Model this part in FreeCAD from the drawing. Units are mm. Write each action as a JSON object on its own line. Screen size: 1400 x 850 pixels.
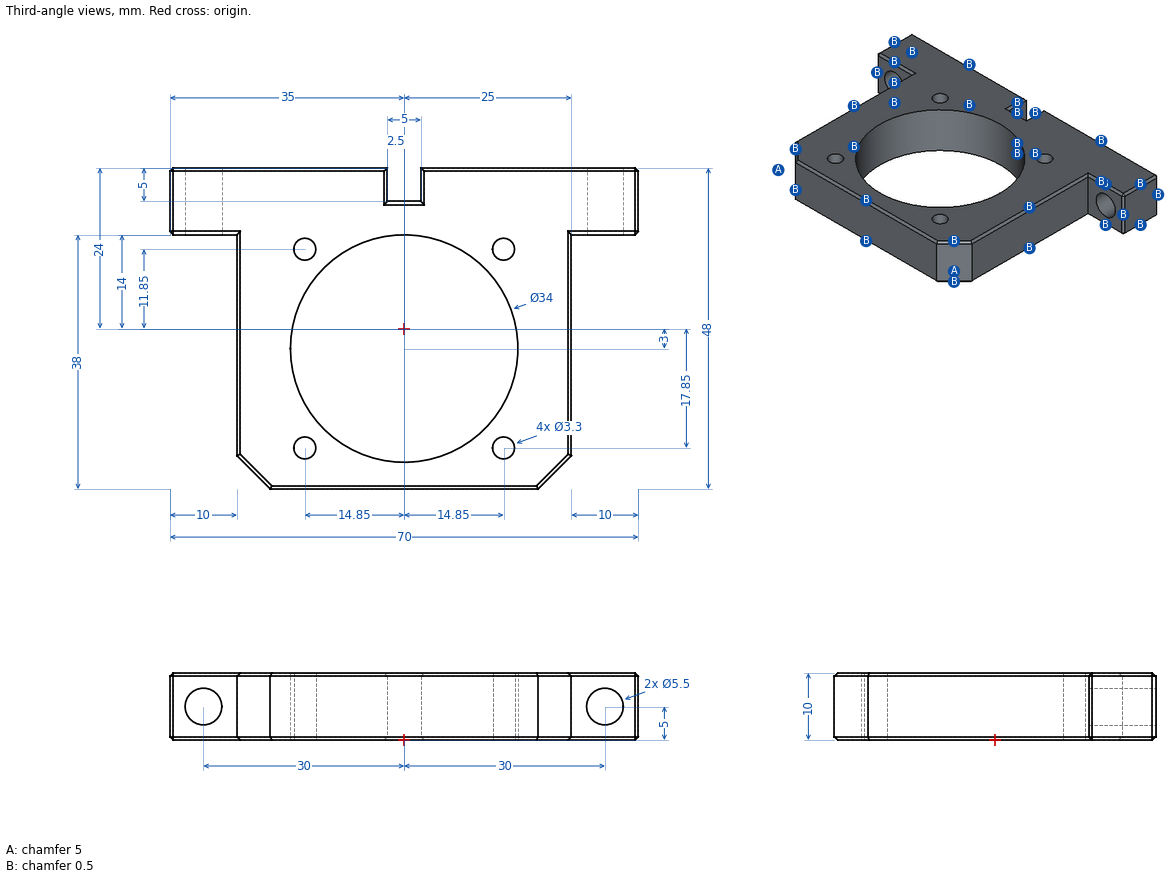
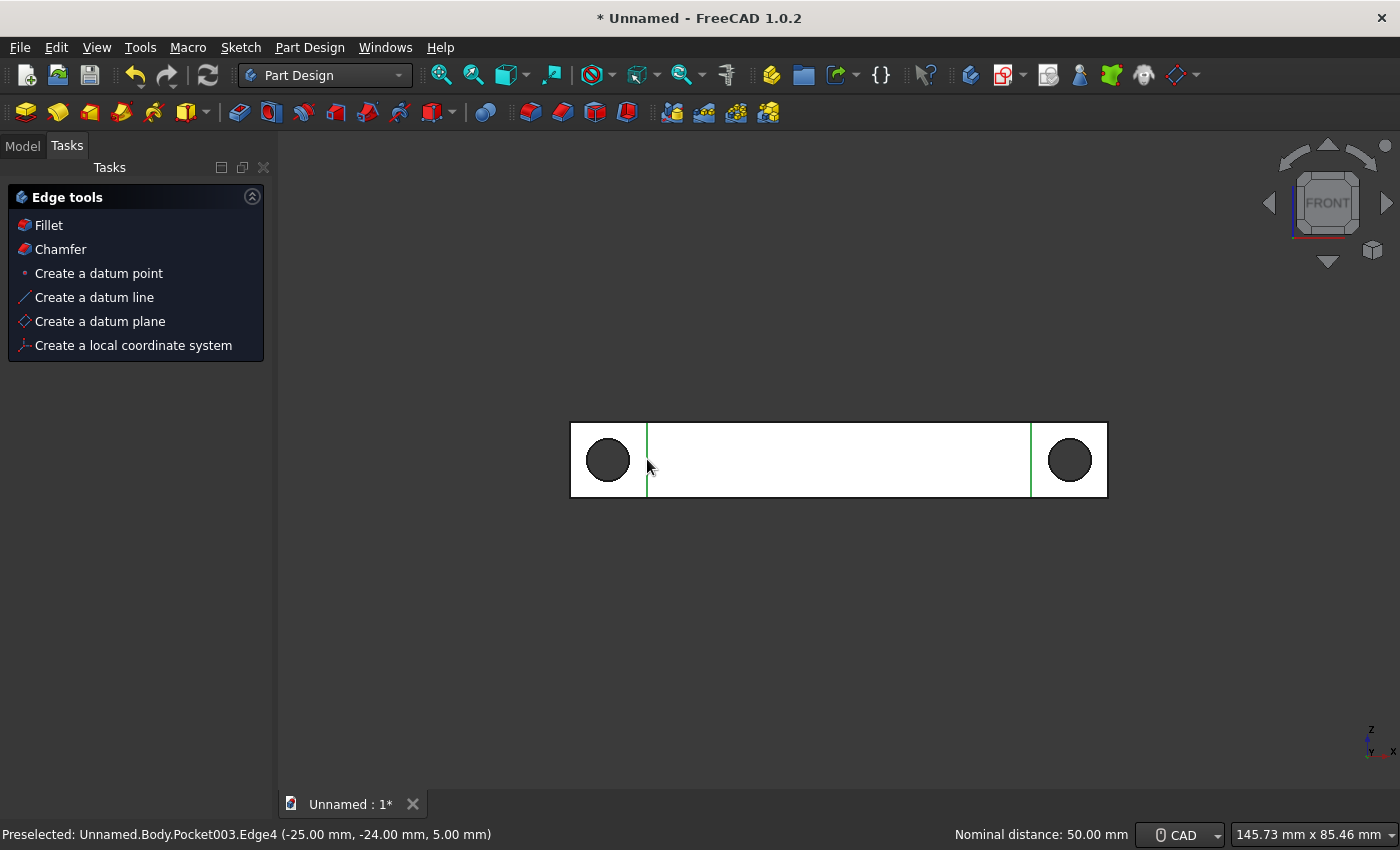
{"action": "left_click", "coordinate": [564, 112]}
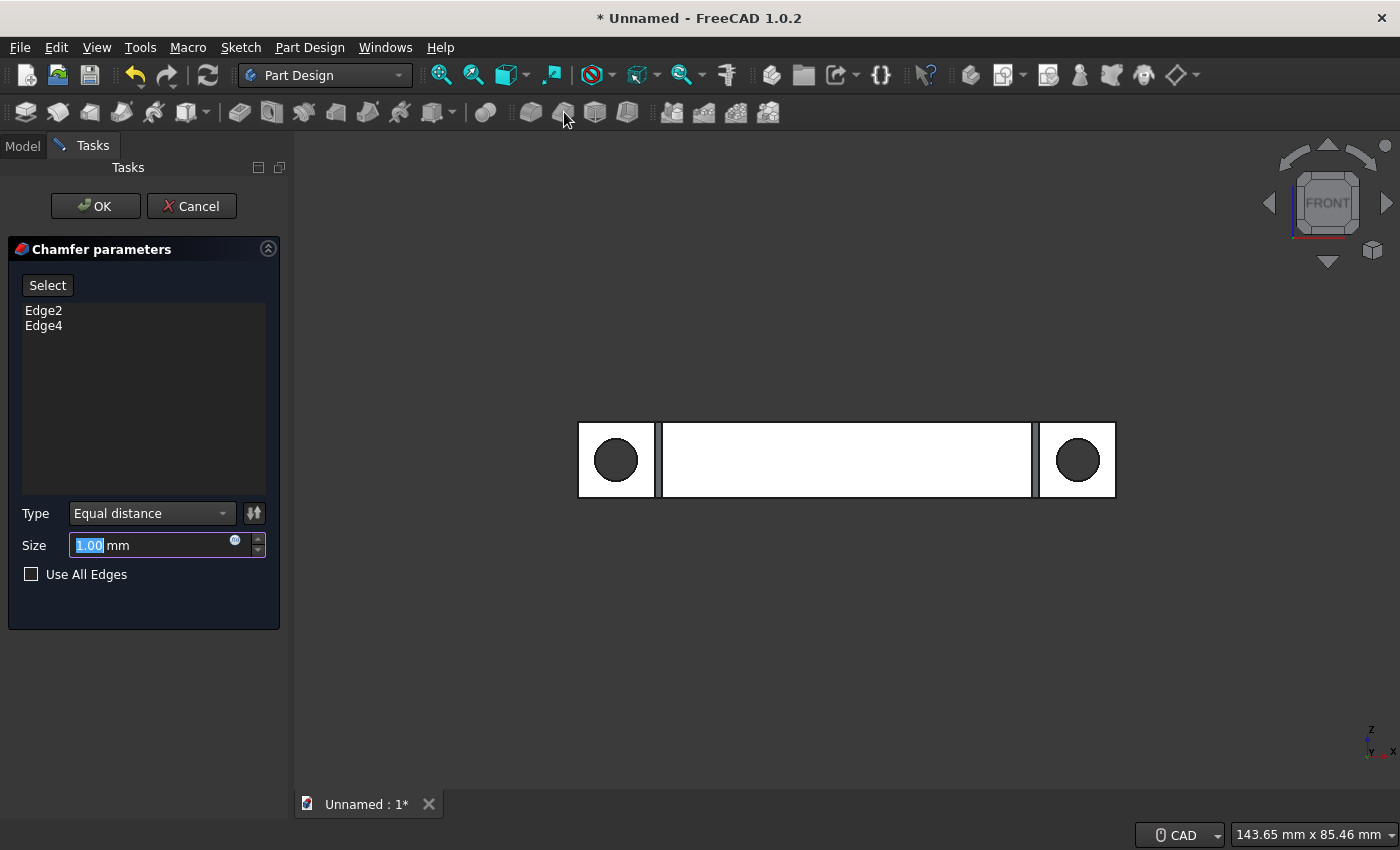
{"action": "type", "text": "5"}
{"action": "key", "text": "Tab"}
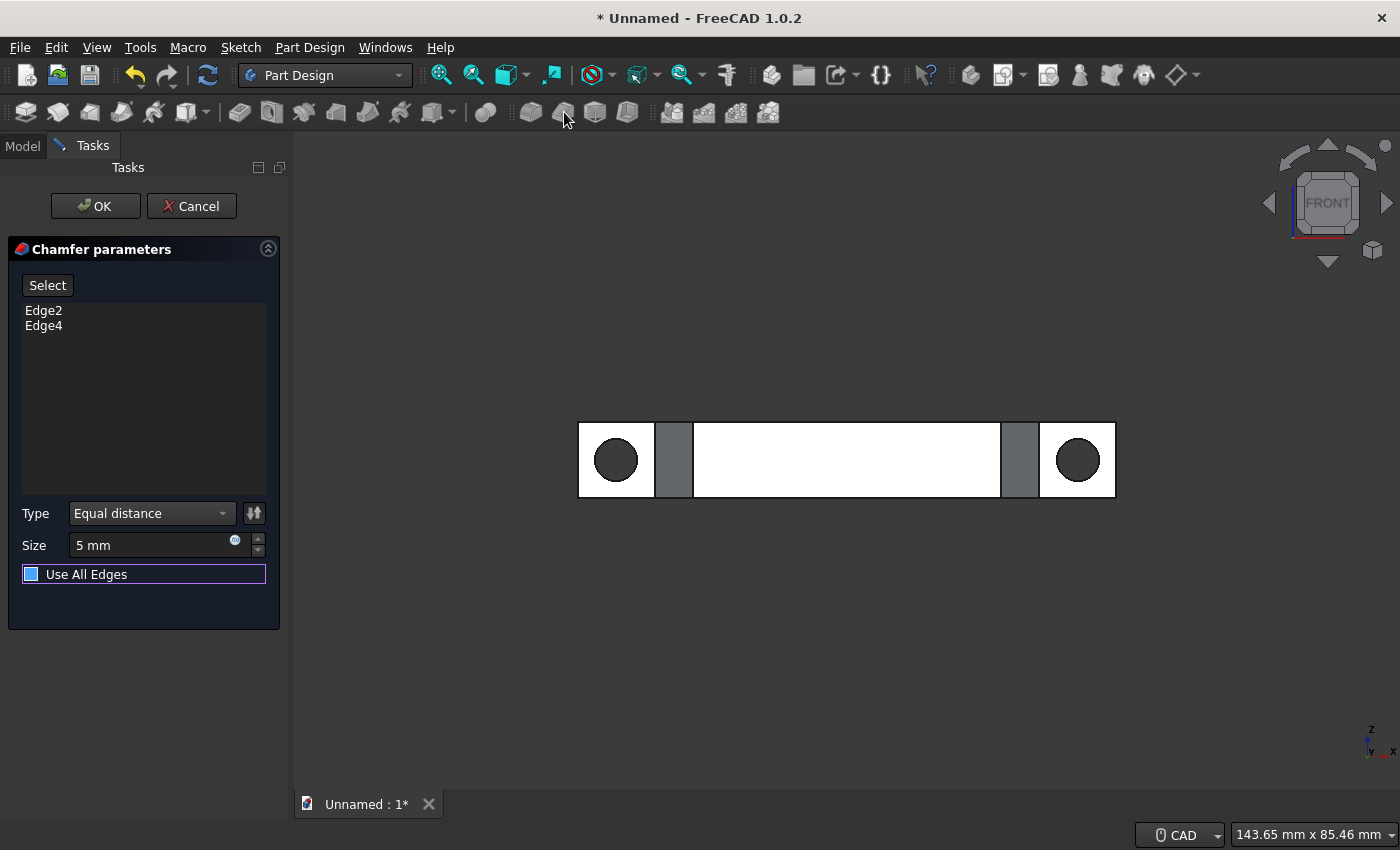
{"action": "left_click", "coordinate": [96, 206]}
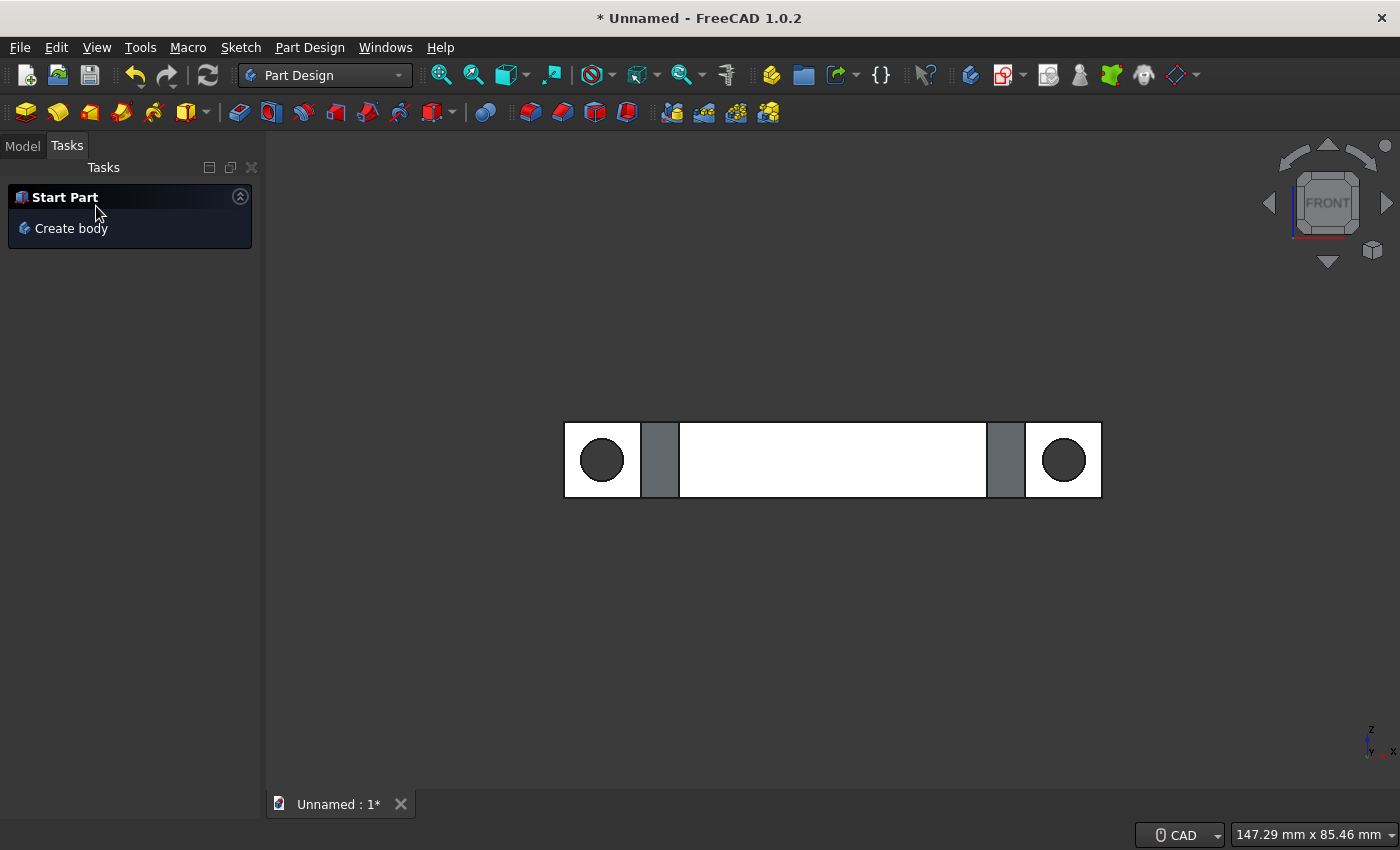
{"action": "key", "text": "0"}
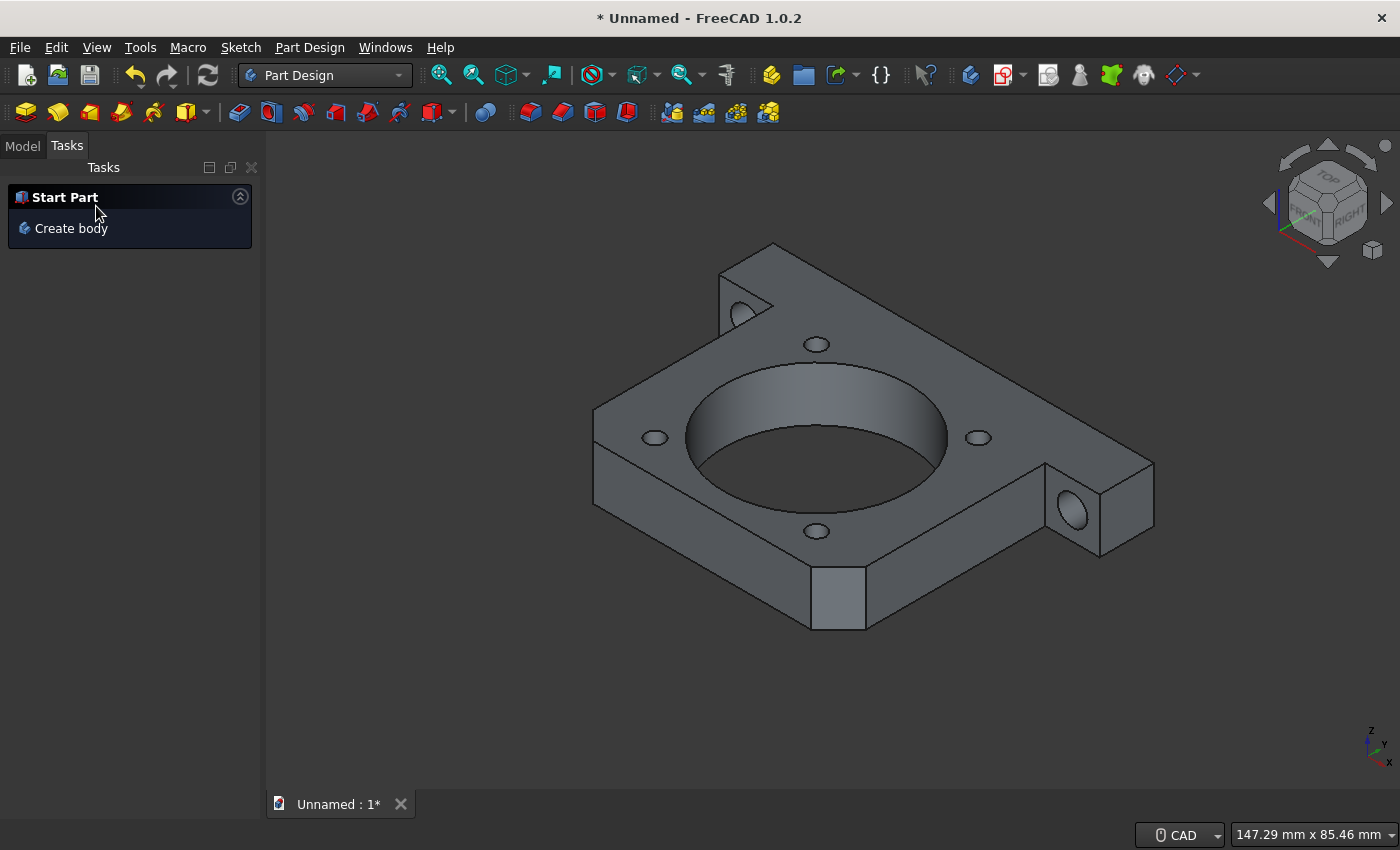
{"action": "left_click", "coordinate": [979, 469]}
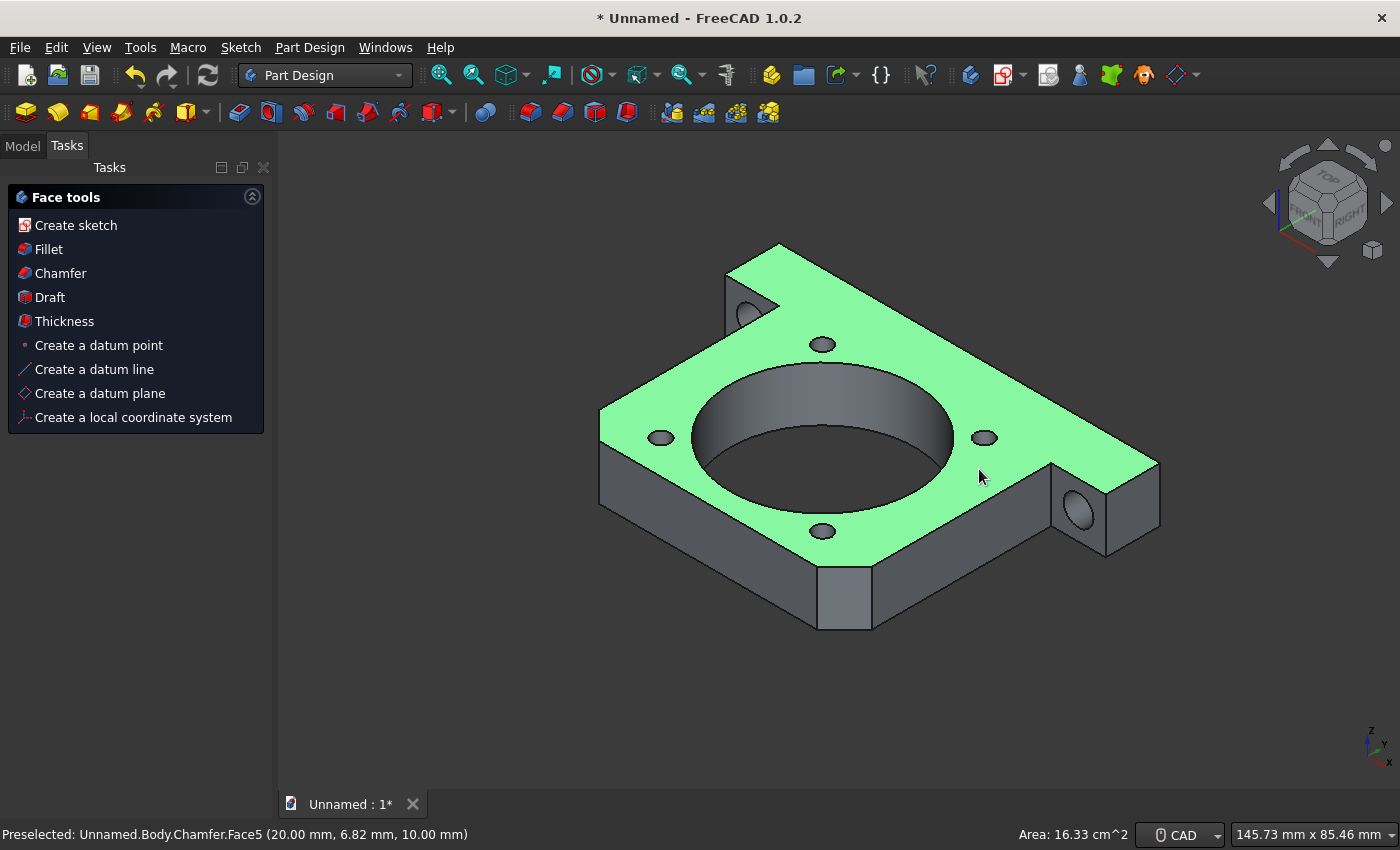
{"action": "left_click", "coordinate": [1004, 76]}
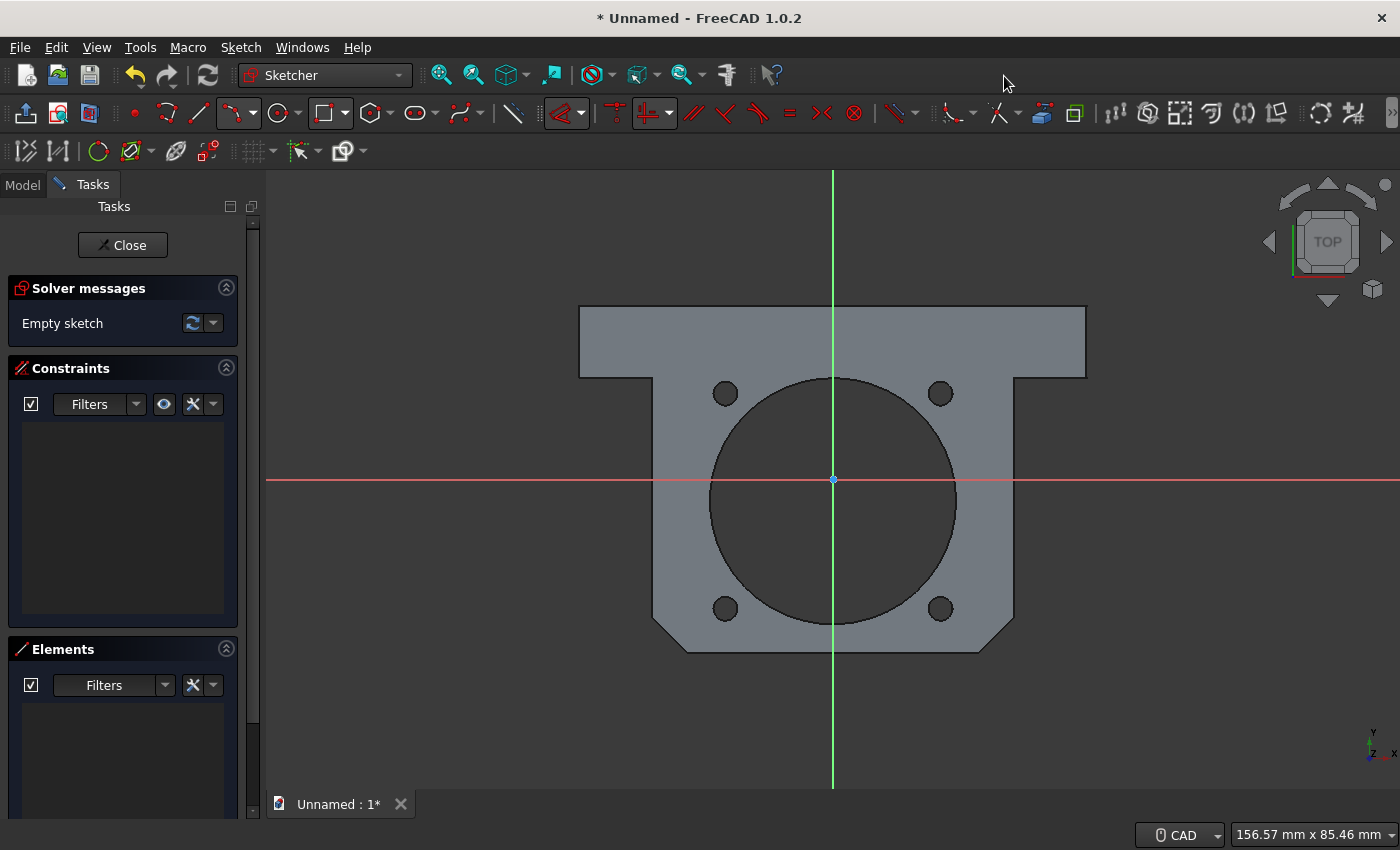
{"action": "scroll", "coordinate": [840, 308], "scroll_direction": "up", "scroll_amount": 12}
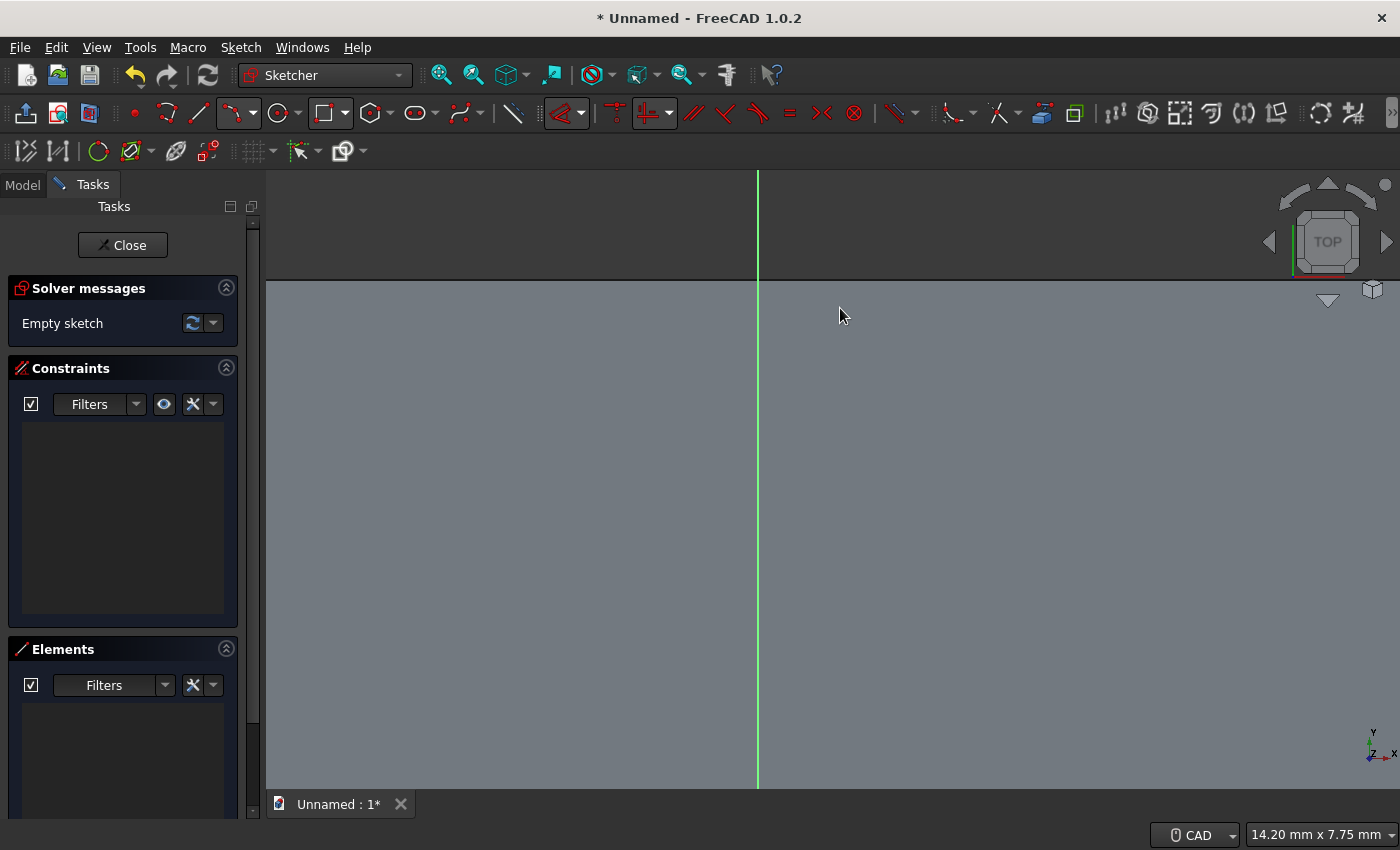
{"action": "left_click", "coordinate": [324, 114]}